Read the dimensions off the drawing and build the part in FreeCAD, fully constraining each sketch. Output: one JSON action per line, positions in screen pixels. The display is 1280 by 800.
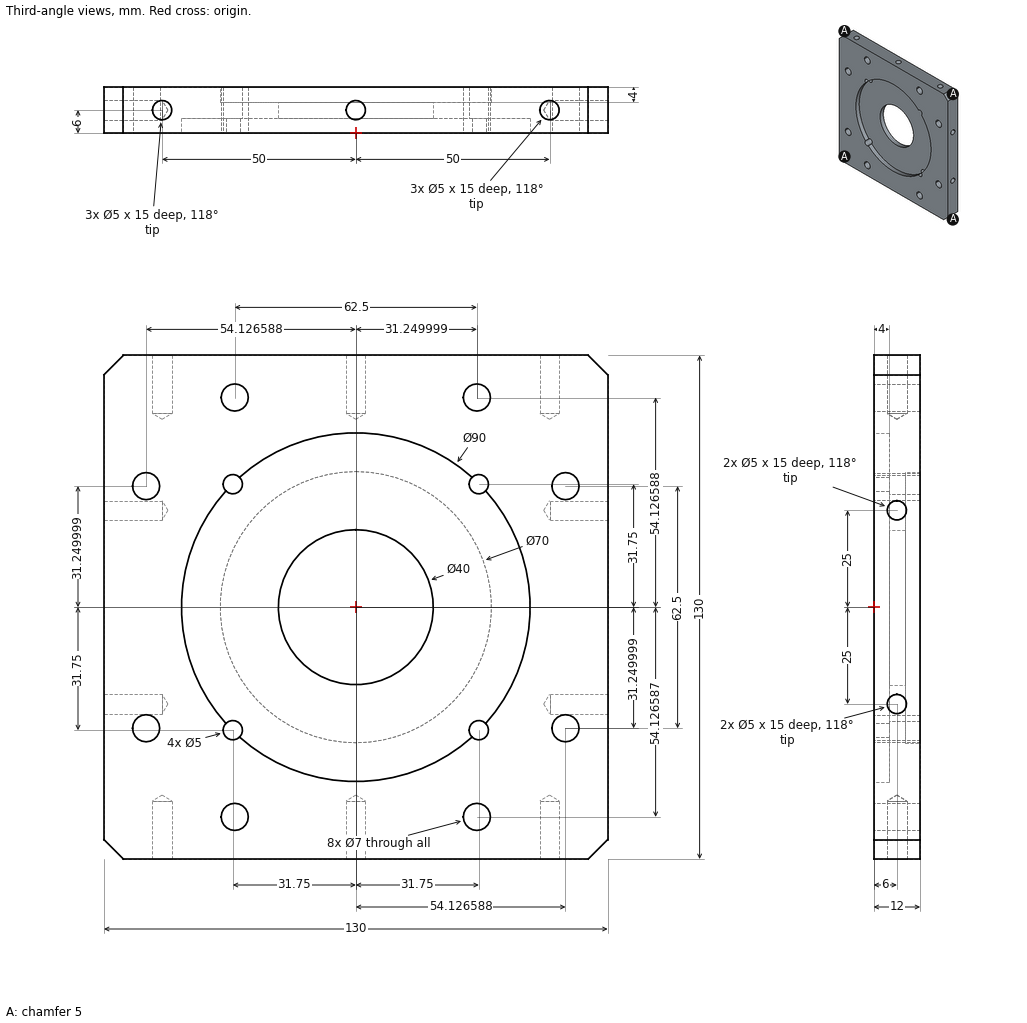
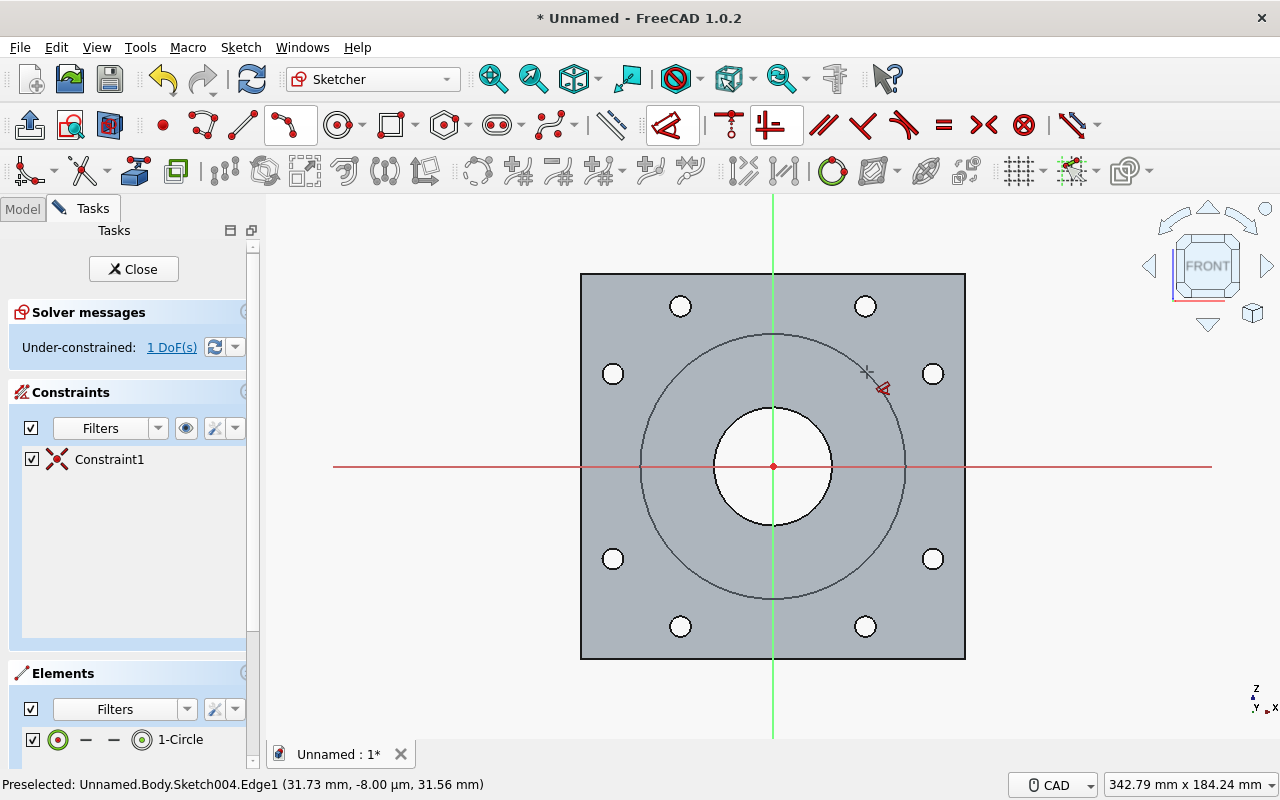
{"action": "left_click", "coordinate": [866, 372]}
{"action": "left_click", "coordinate": [888, 349]}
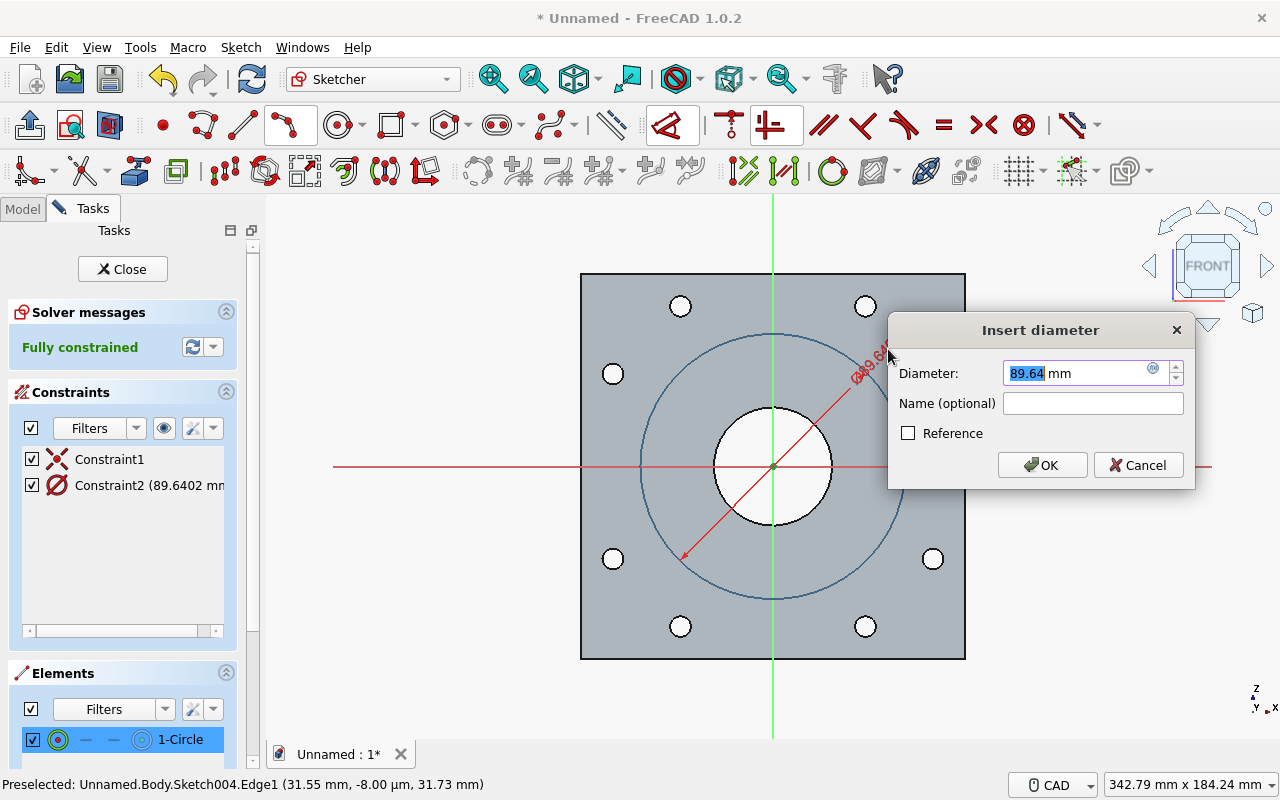
{"action": "type", "text": "90"}
{"action": "key", "text": "Return"}
{"action": "key", "text": "Escape"}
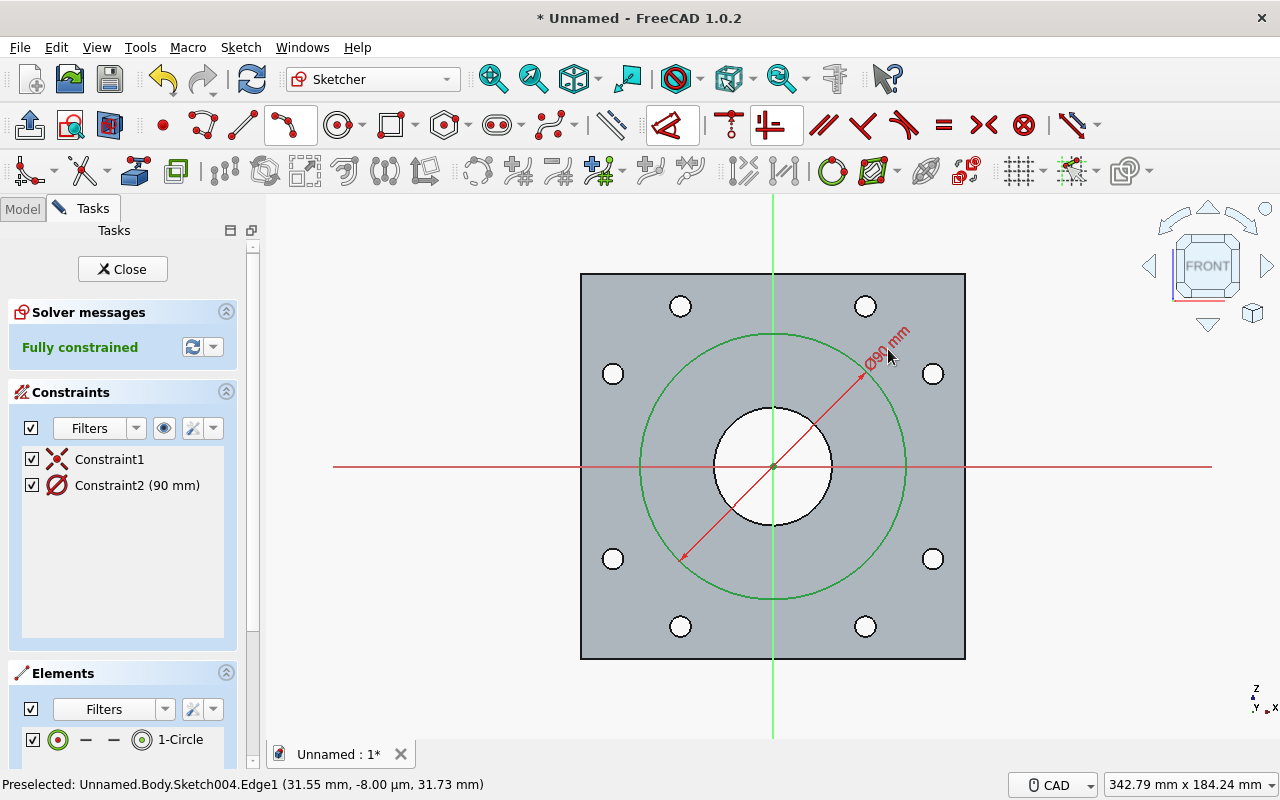
{"action": "left_click", "coordinate": [123, 269]}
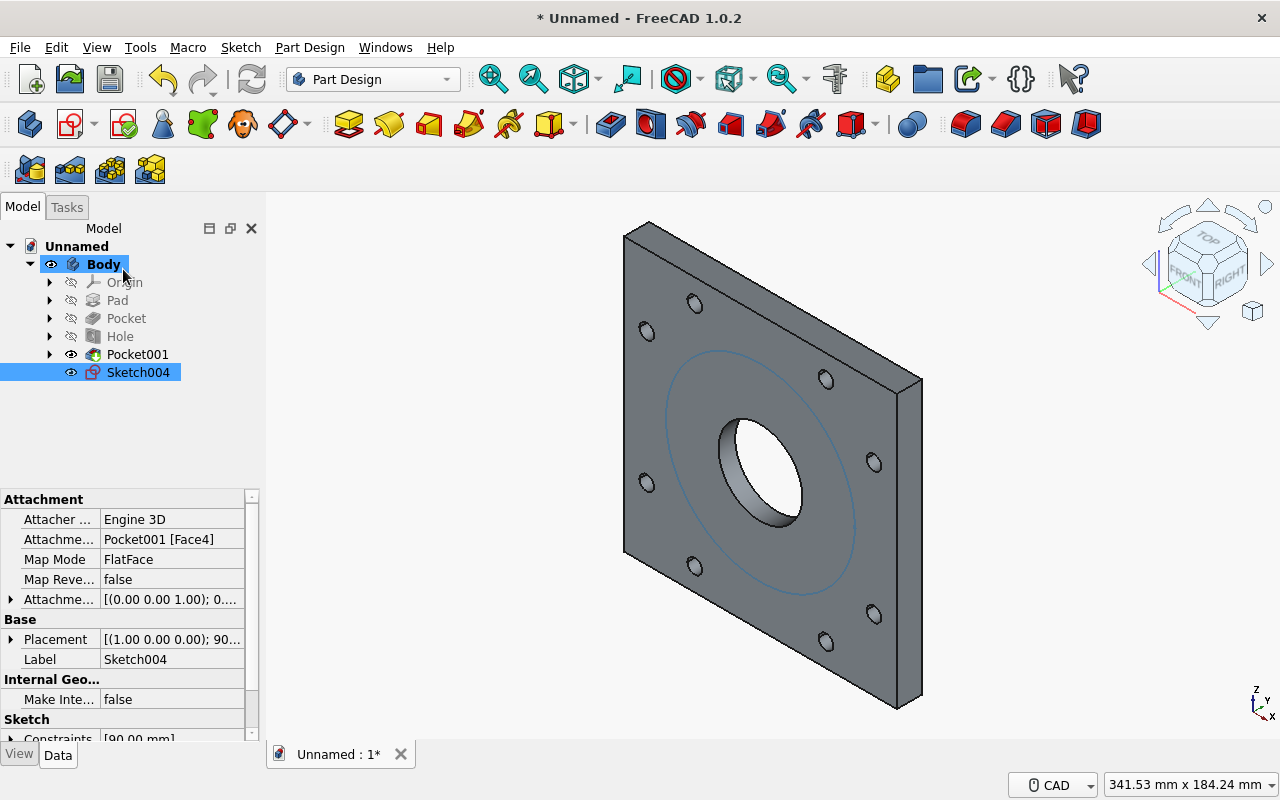
{"action": "left_click", "coordinate": [612, 124]}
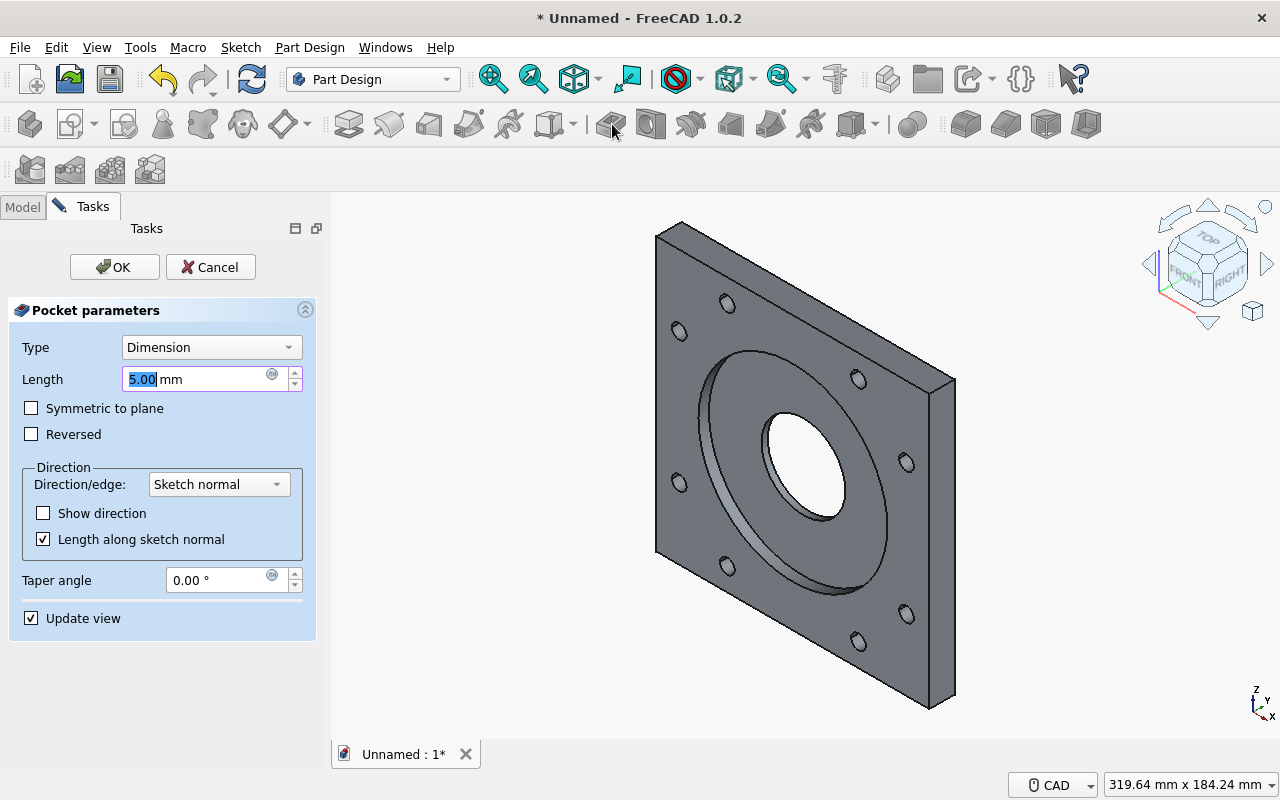
{"action": "type", "text": "4"}
{"action": "key", "text": "Tab"}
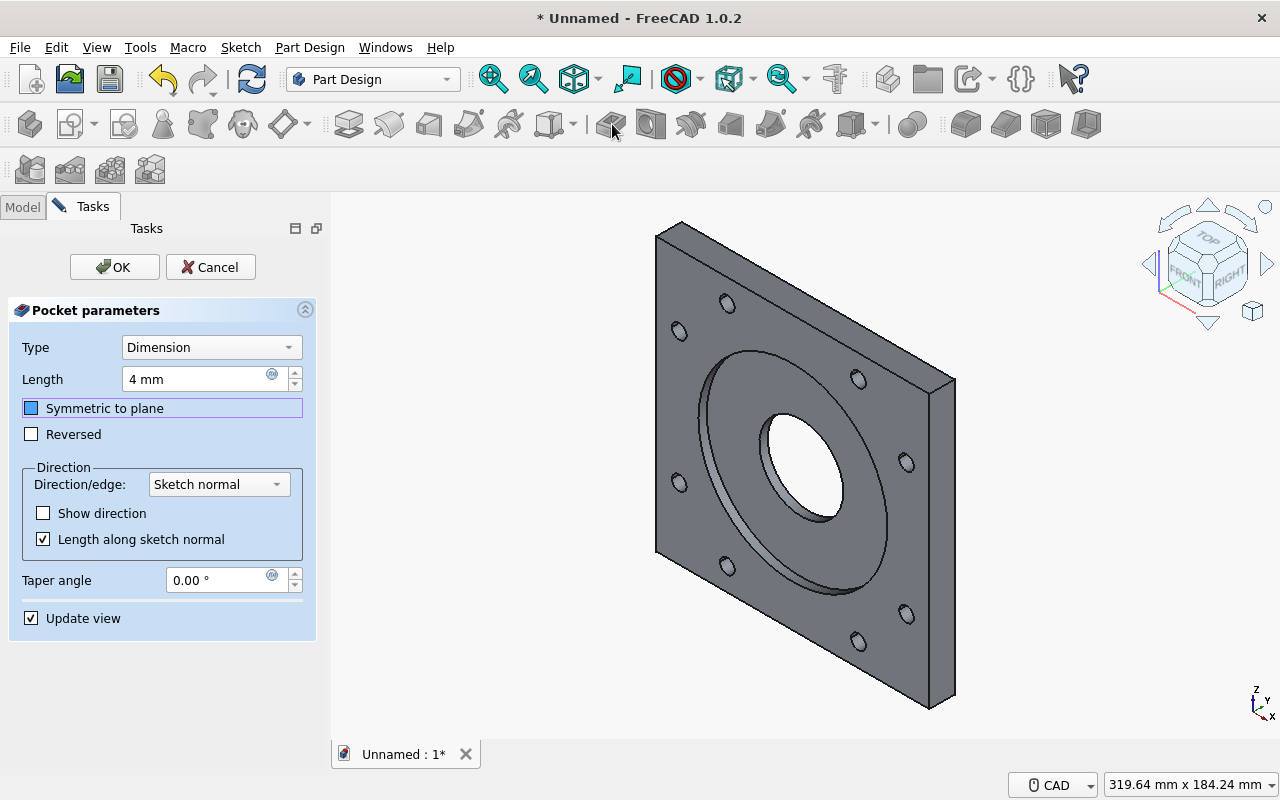
{"action": "left_click", "coordinate": [115, 267]}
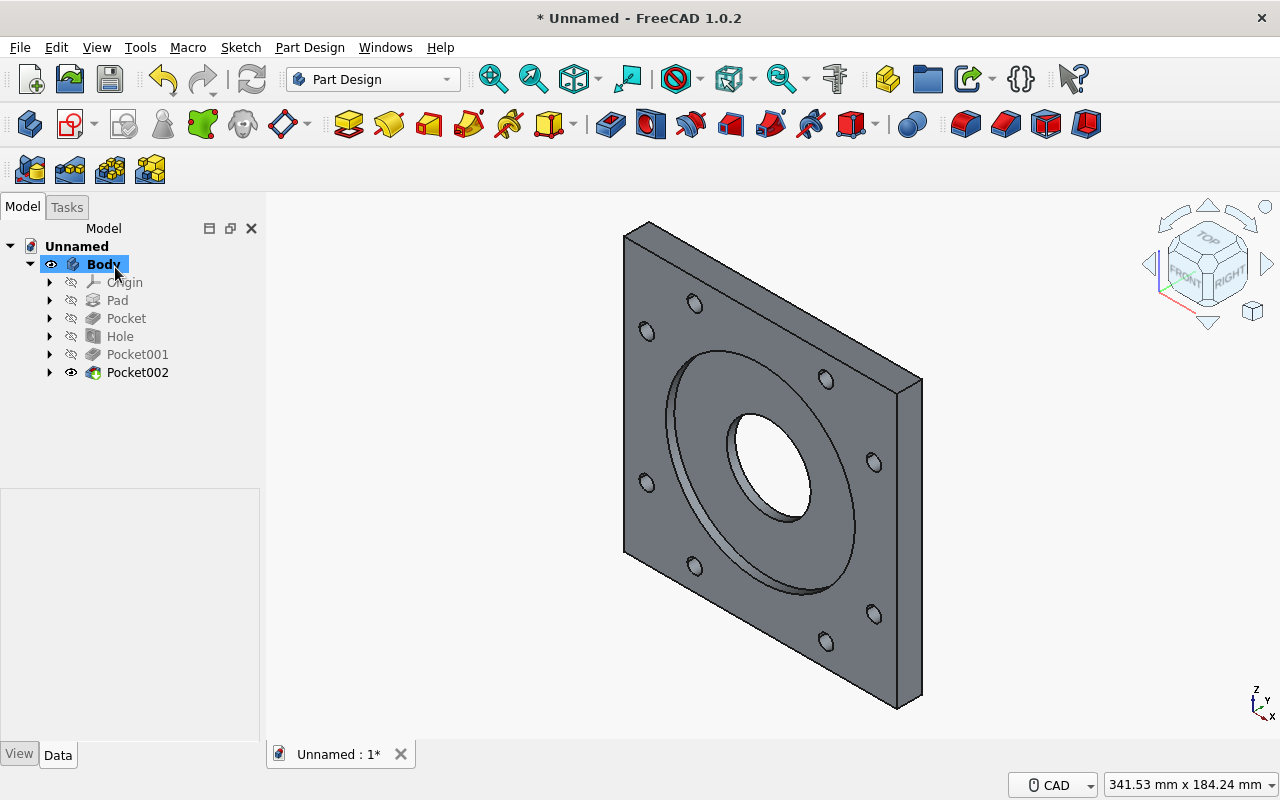
{"action": "key", "text": "4"}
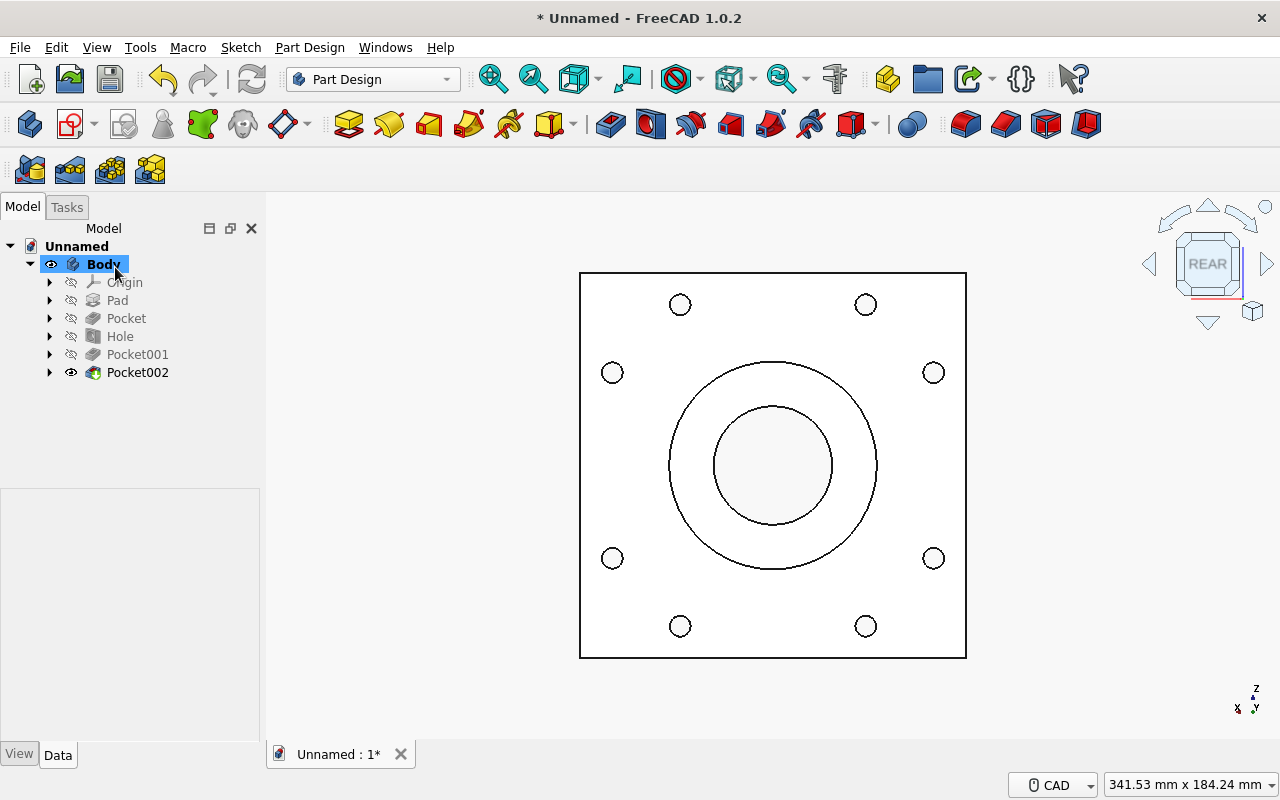
{"action": "left_click", "coordinate": [663, 354]}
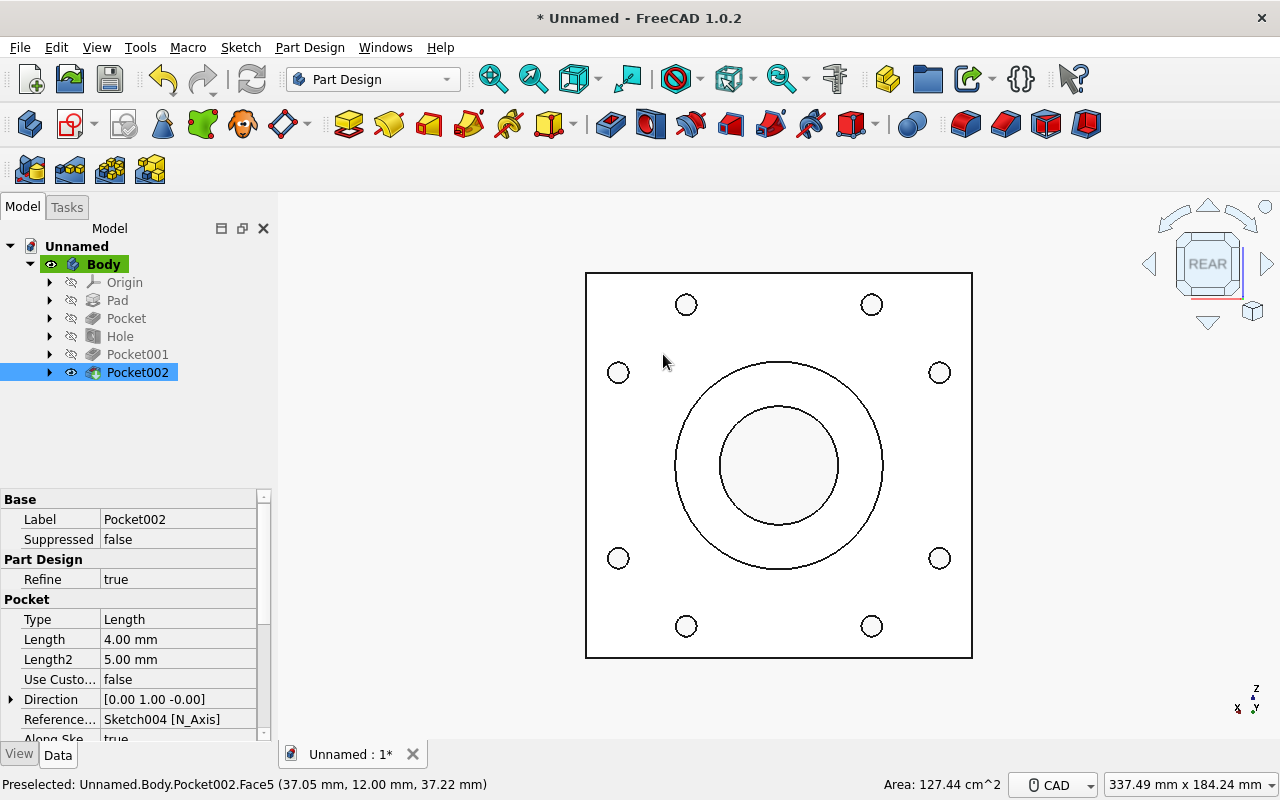
{"action": "left_click", "coordinate": [70, 124]}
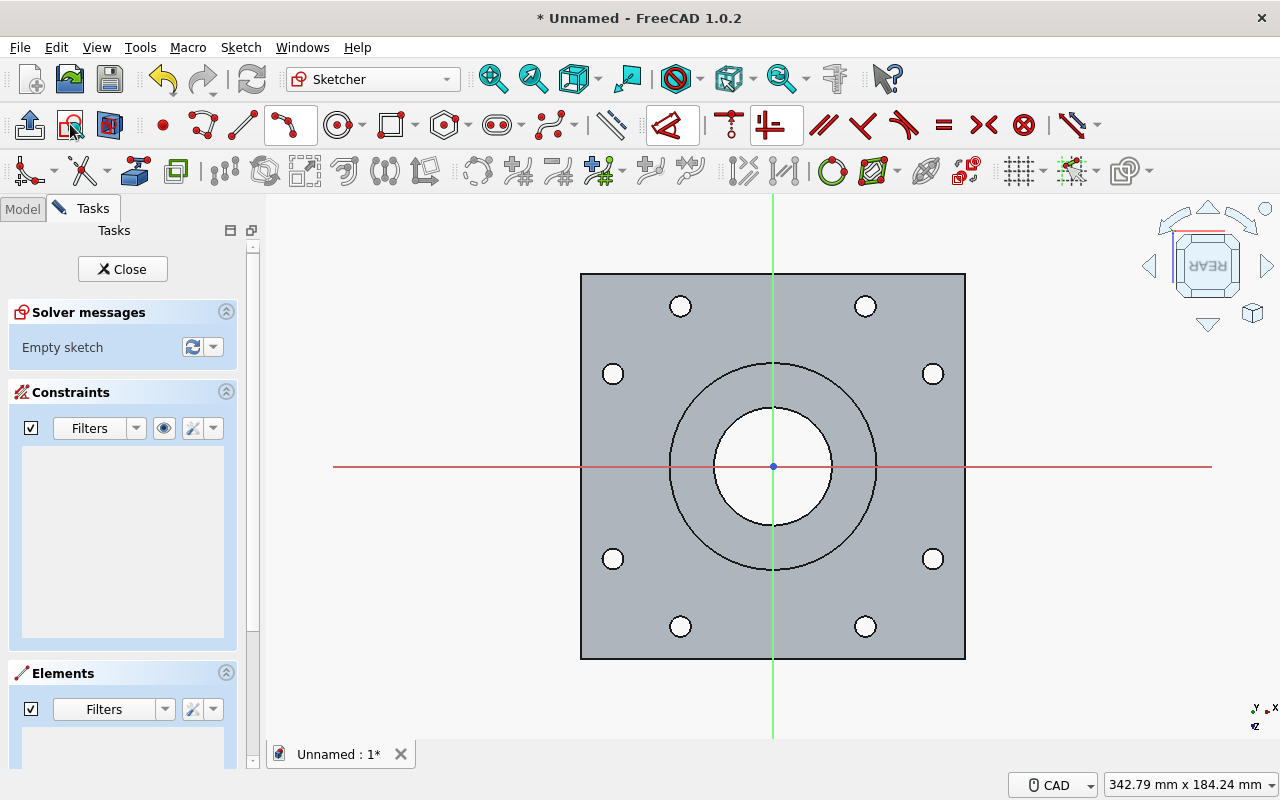
{"action": "scroll", "coordinate": [856, 466], "scroll_direction": "up", "scroll_amount": 3}